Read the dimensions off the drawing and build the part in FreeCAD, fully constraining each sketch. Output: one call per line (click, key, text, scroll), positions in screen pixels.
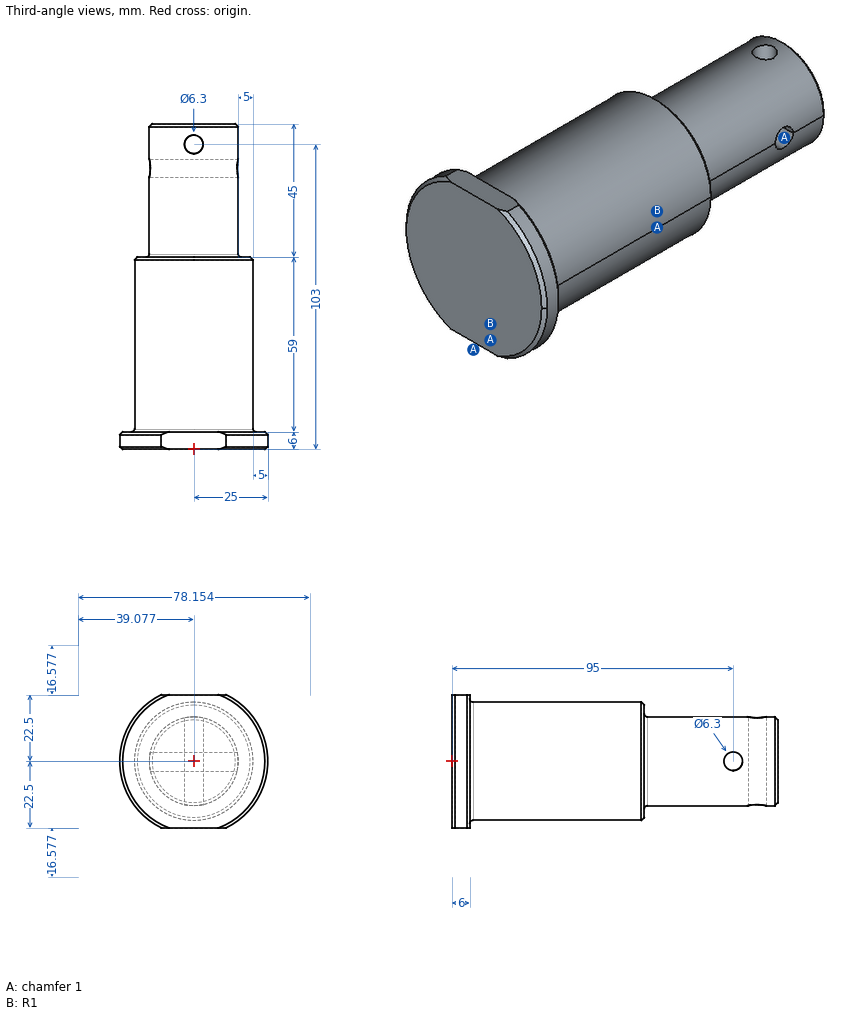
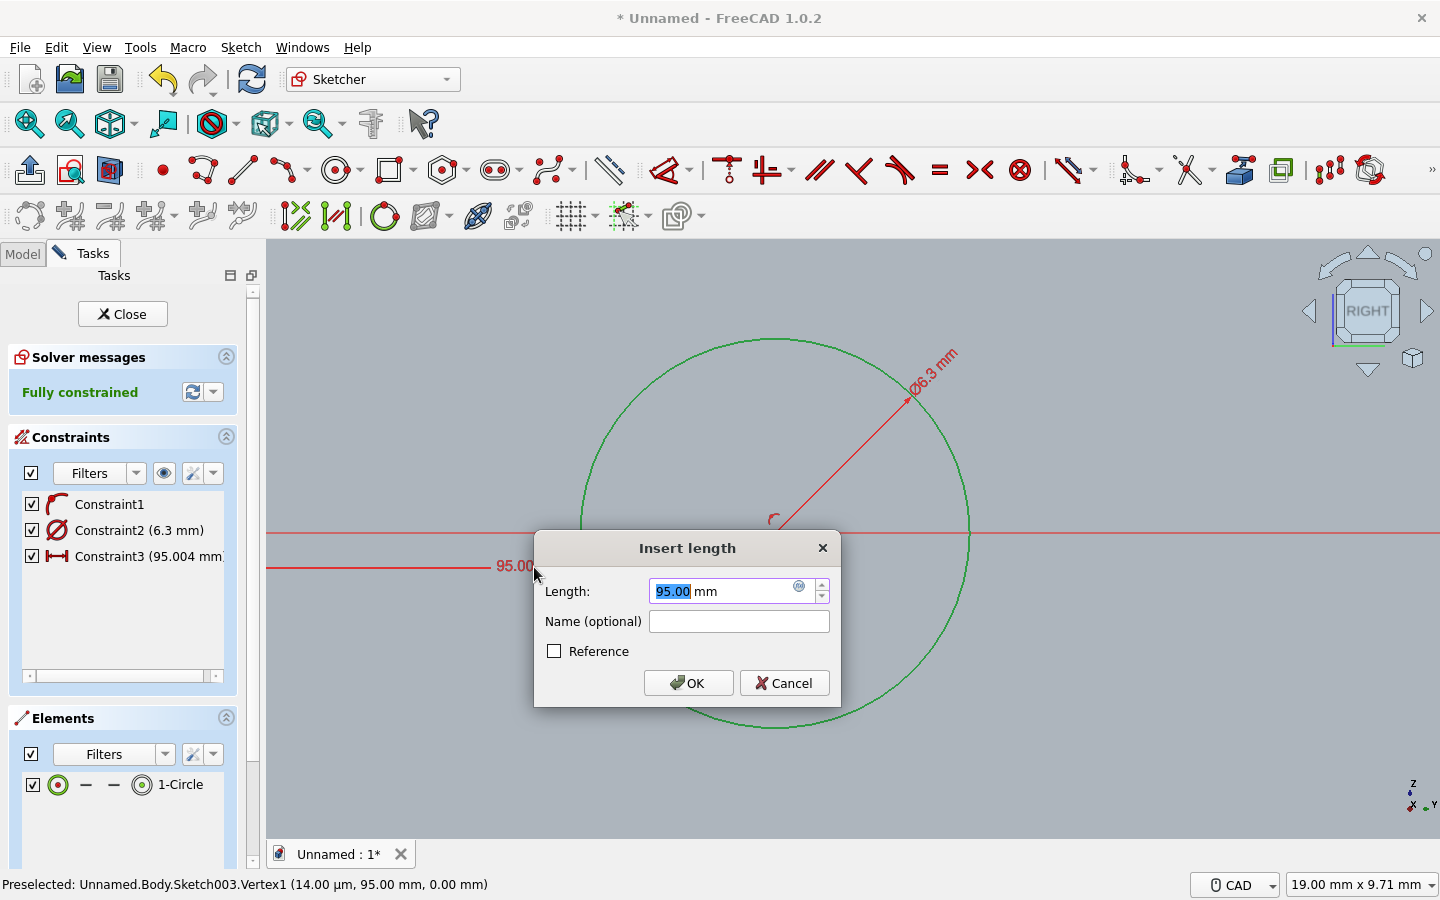
text(95)
key(Return)
key(Escape)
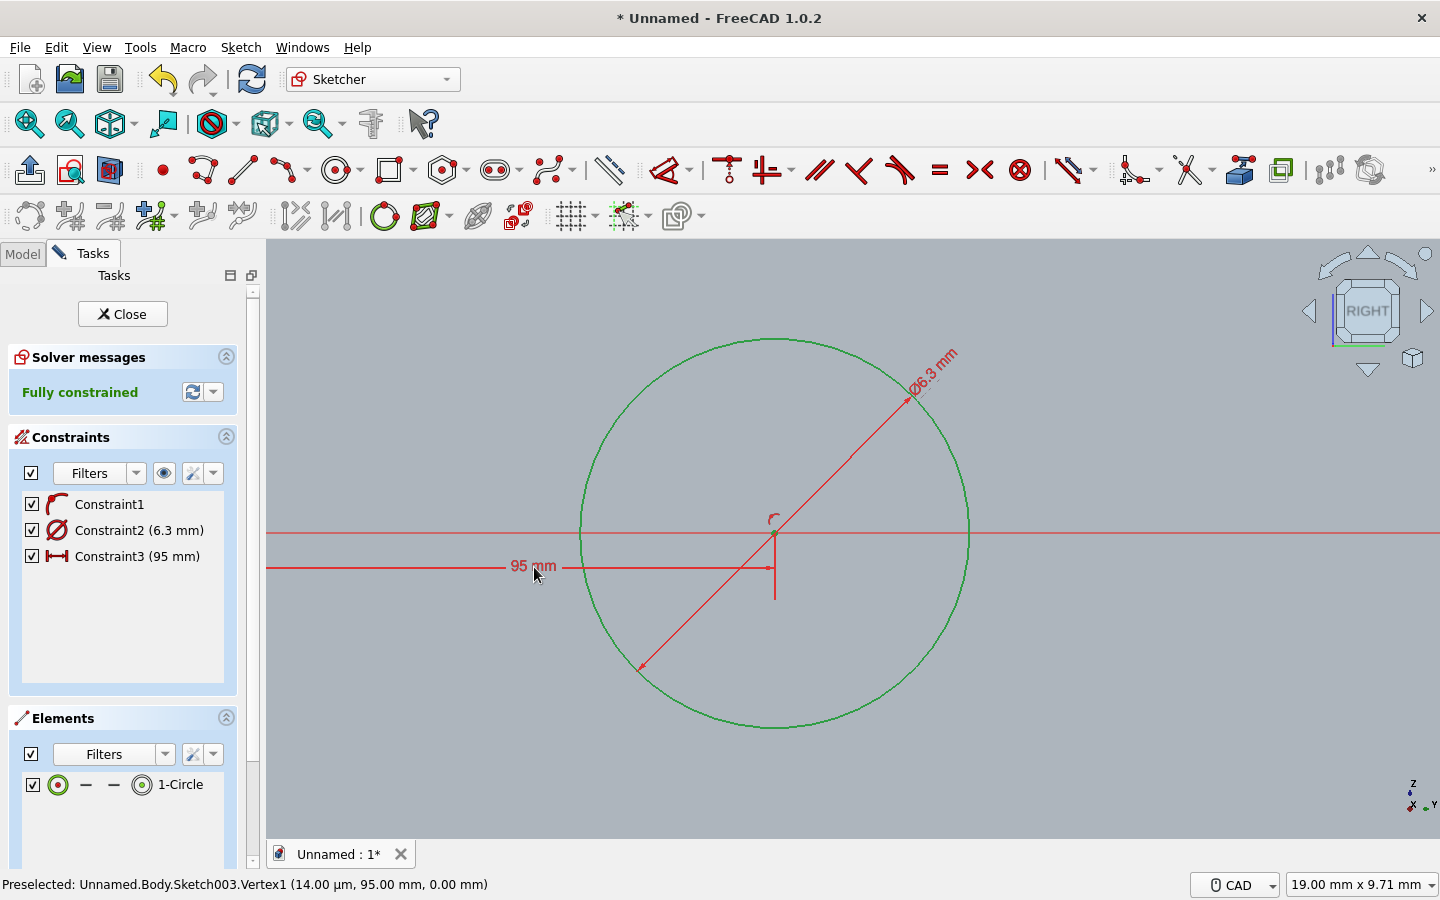
click(123, 314)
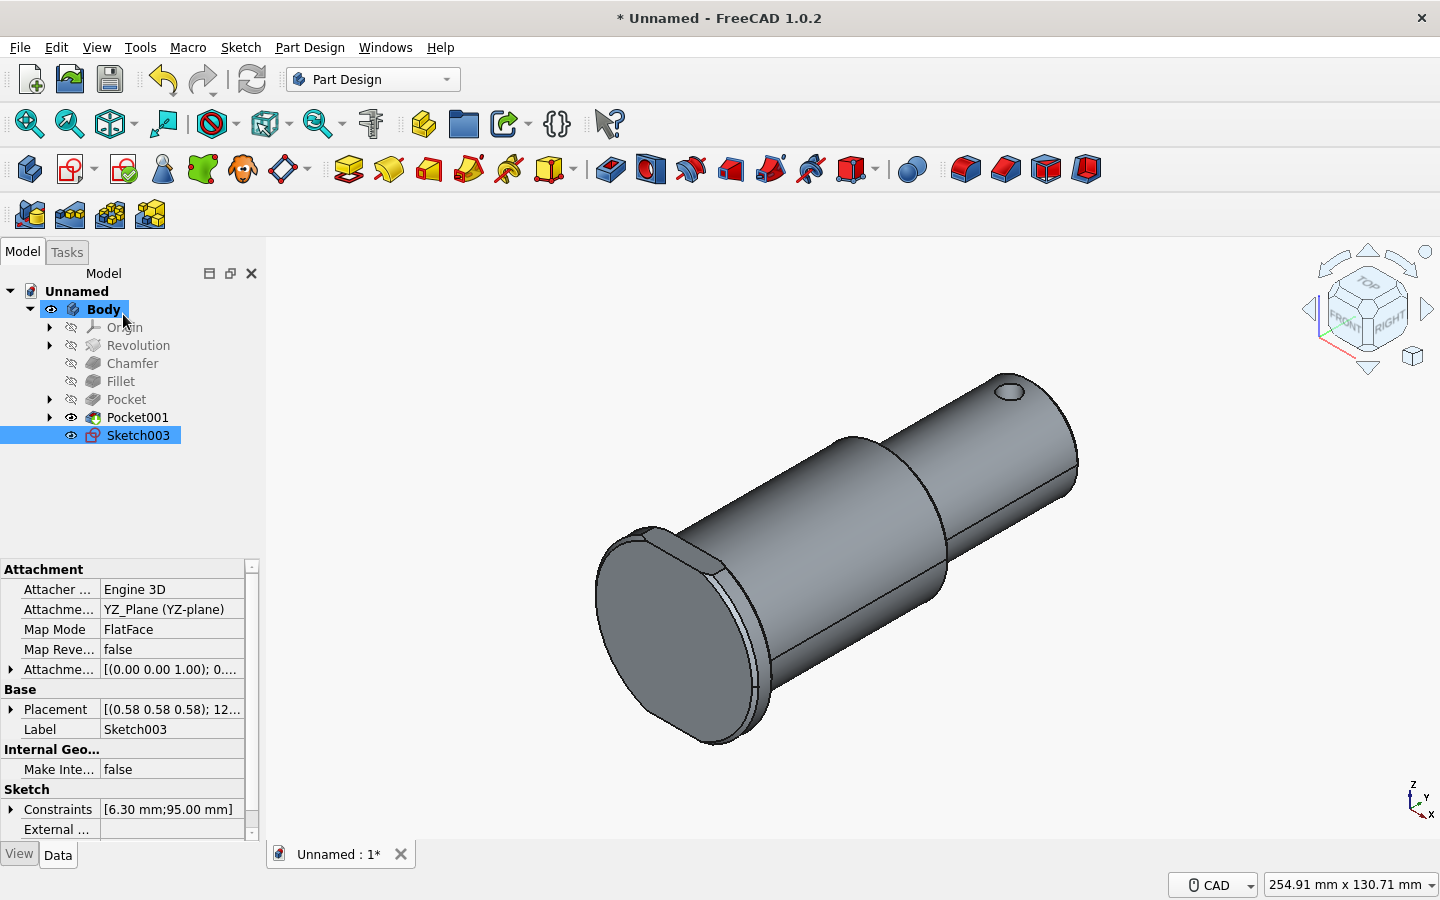
click(612, 170)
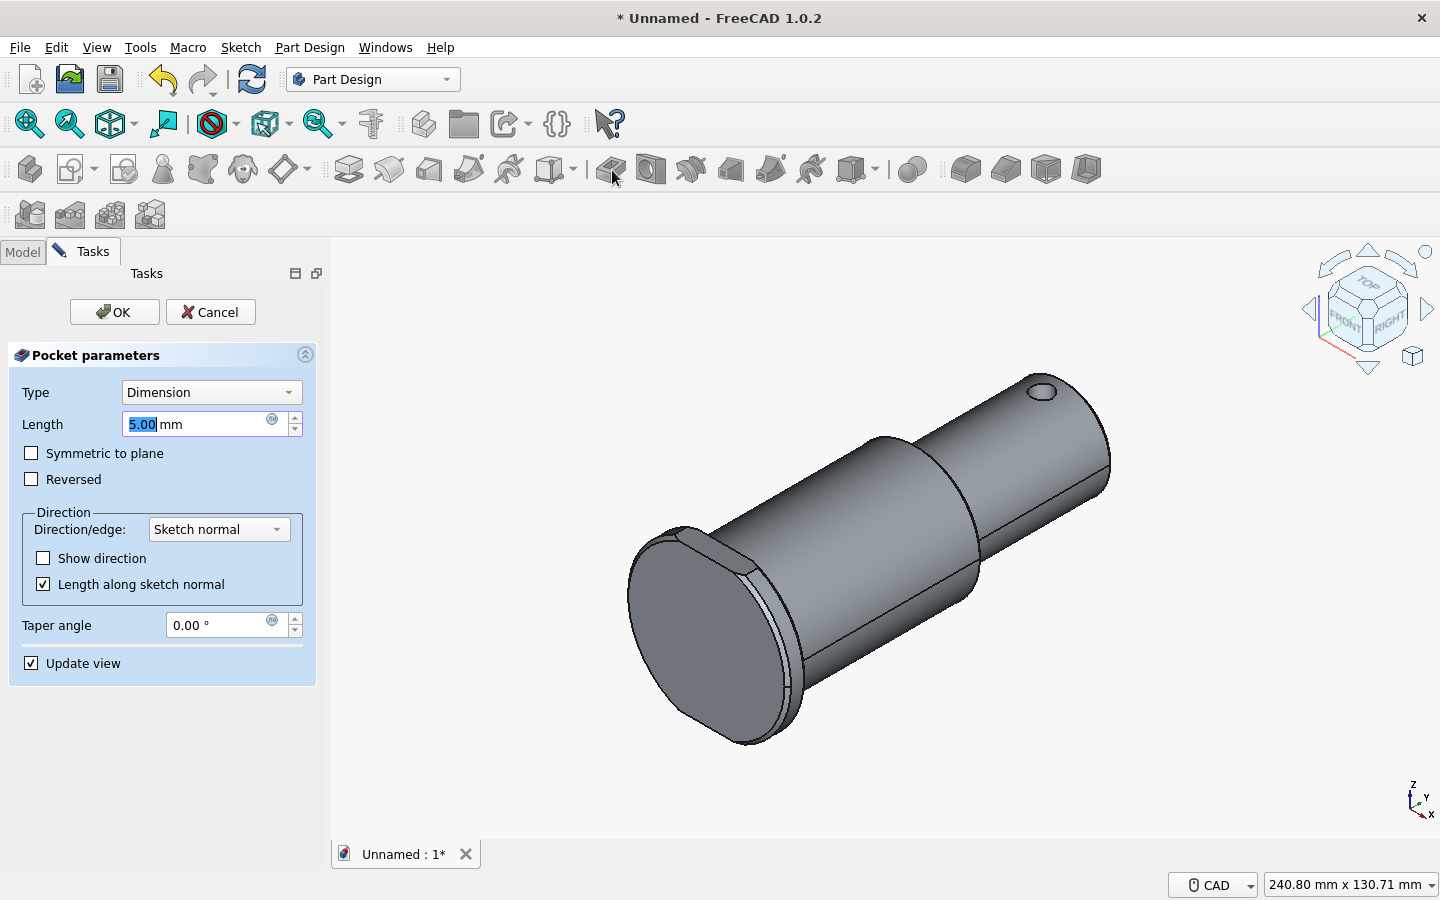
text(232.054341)
key(Tab)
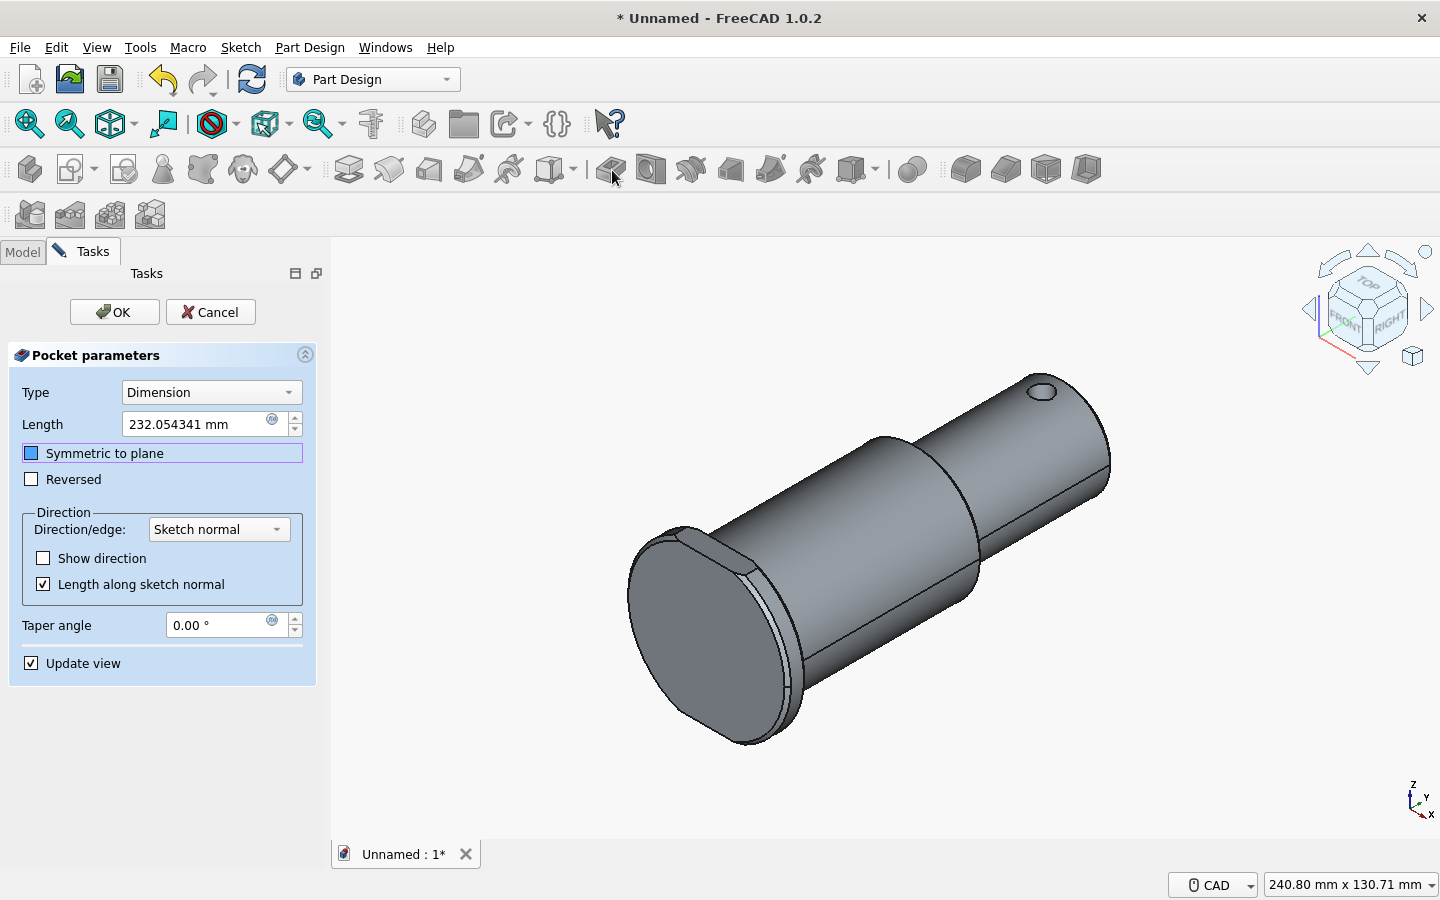
click(30, 453)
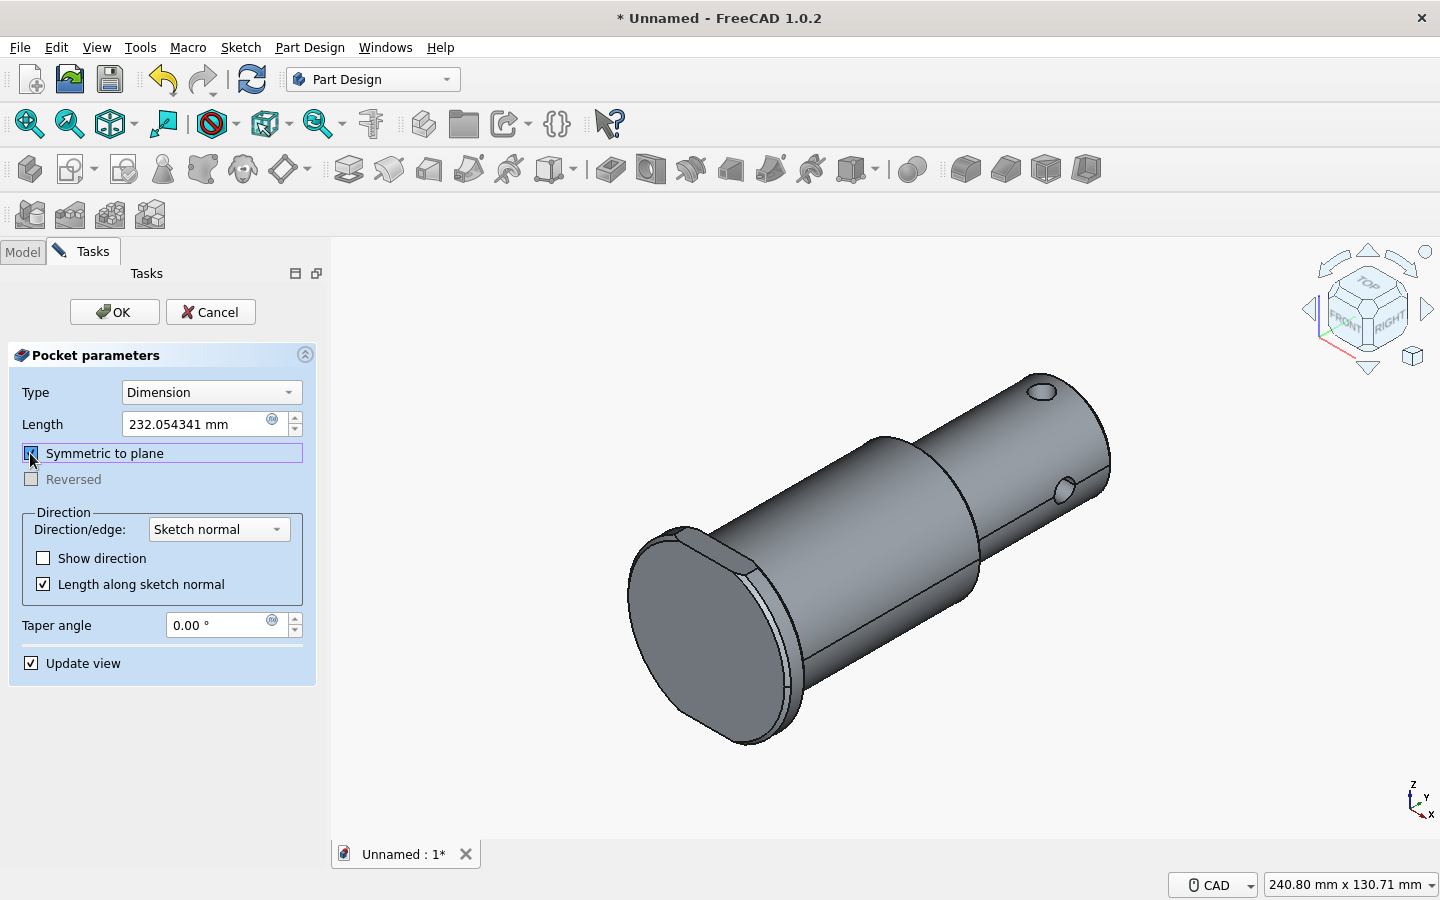
click(115, 312)